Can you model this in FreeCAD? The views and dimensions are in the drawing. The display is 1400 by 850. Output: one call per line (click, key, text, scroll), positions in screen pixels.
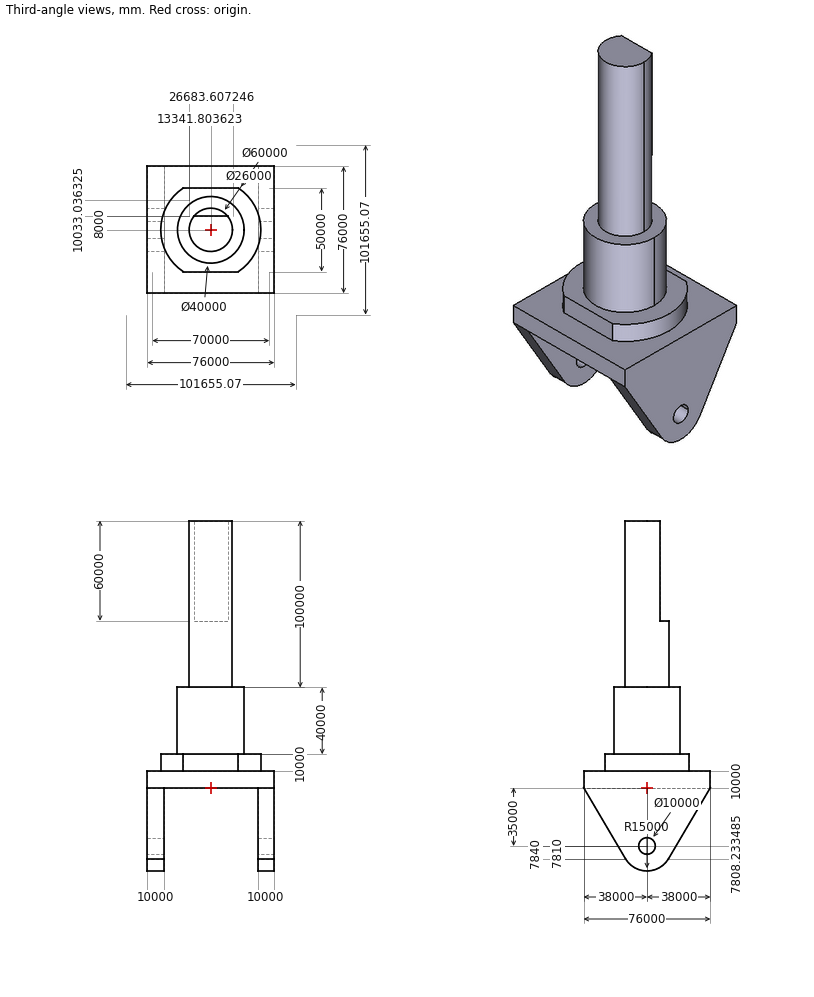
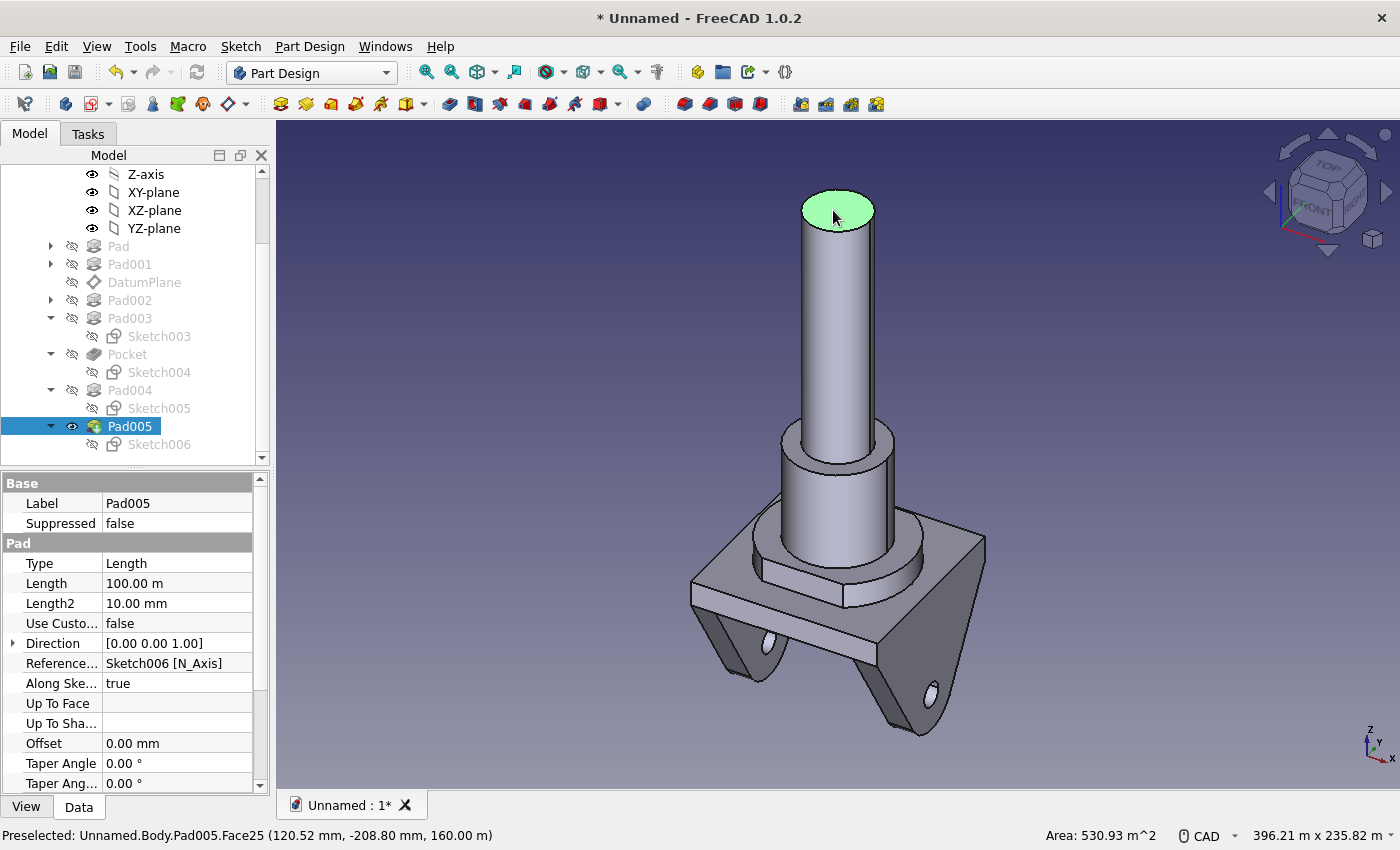
click(90, 104)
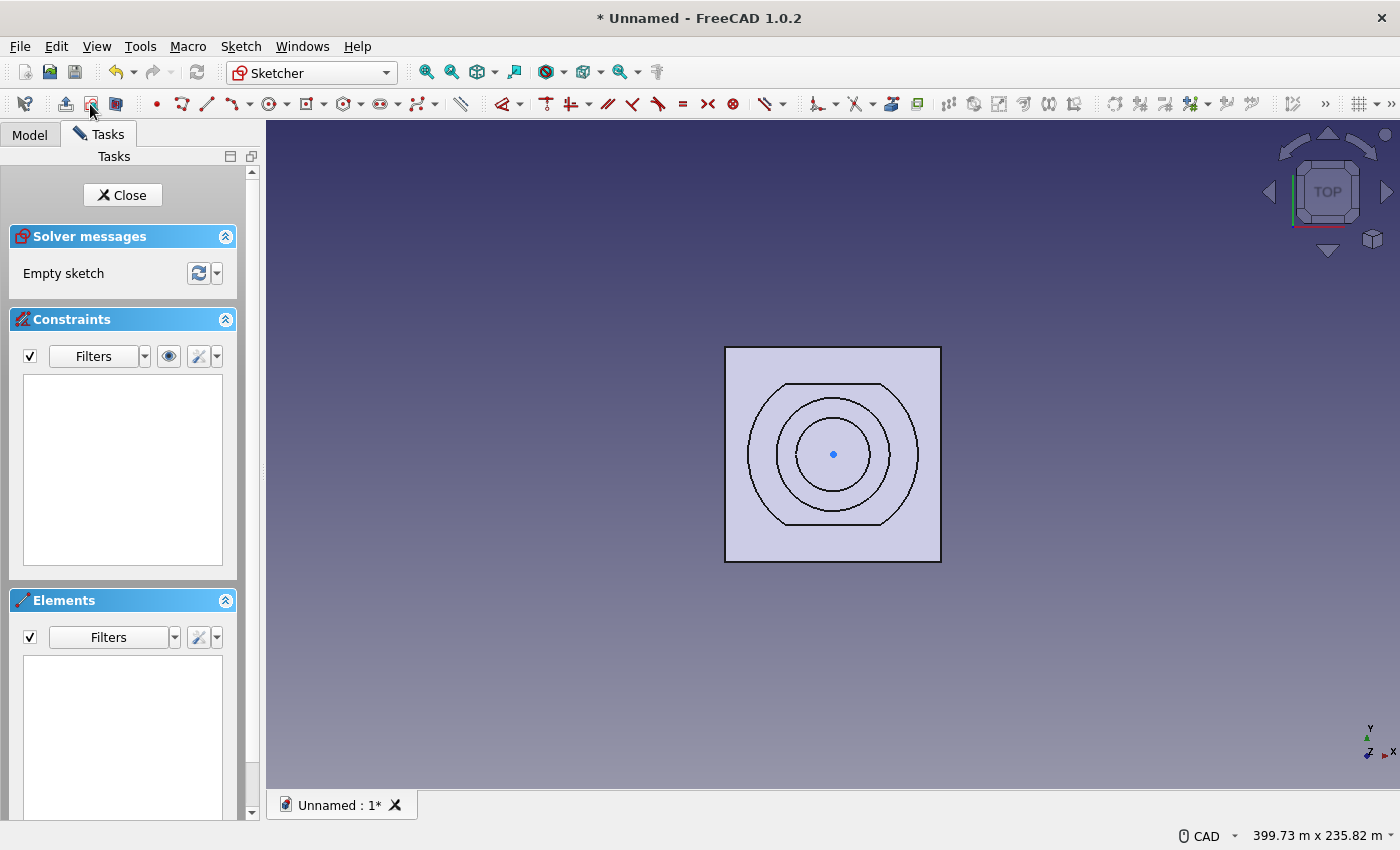
scroll(842, 426, up, 11)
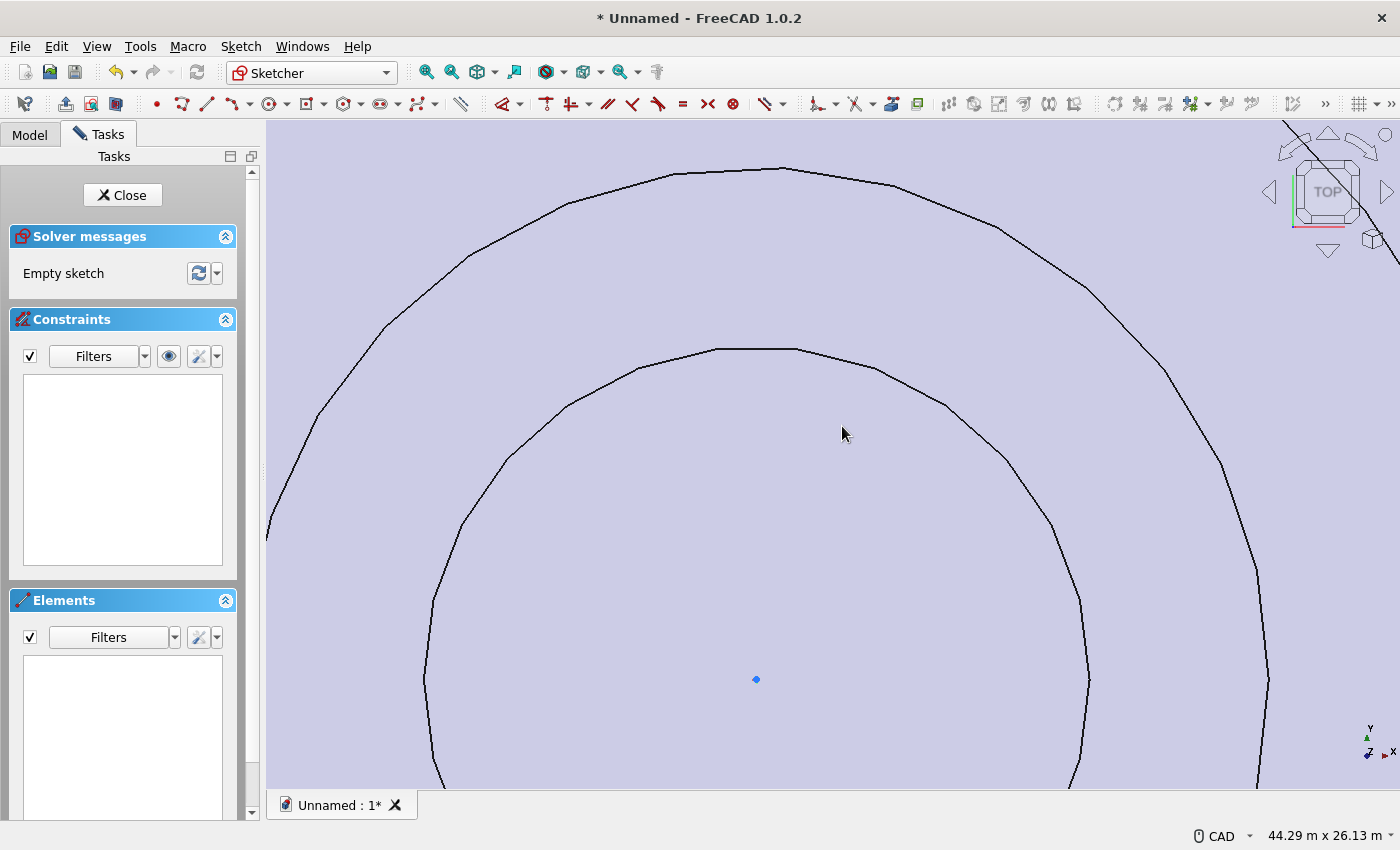
key(g)
key(r)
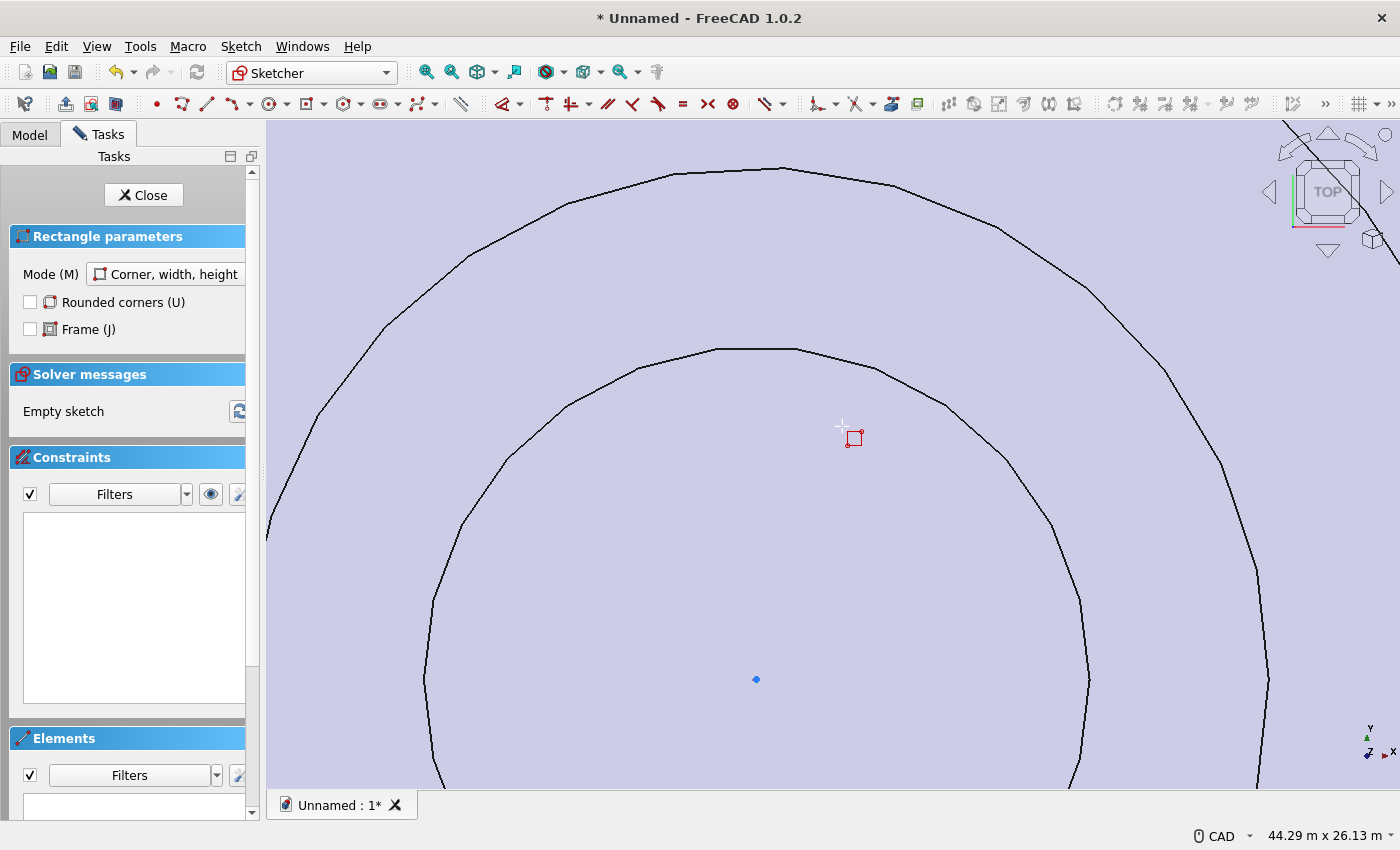
click(415, 218)
click(1098, 475)
key(Escape)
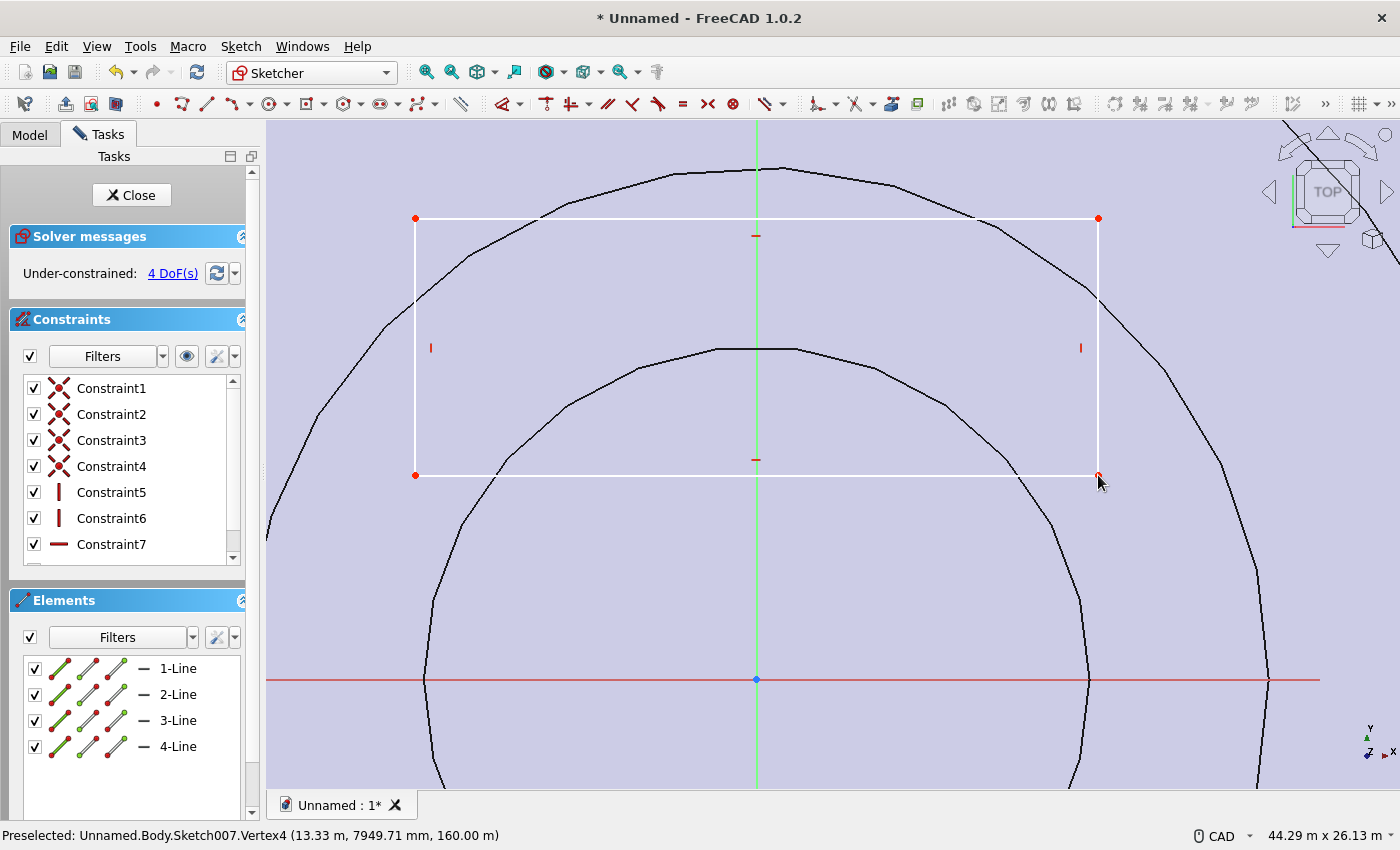
click(502, 104)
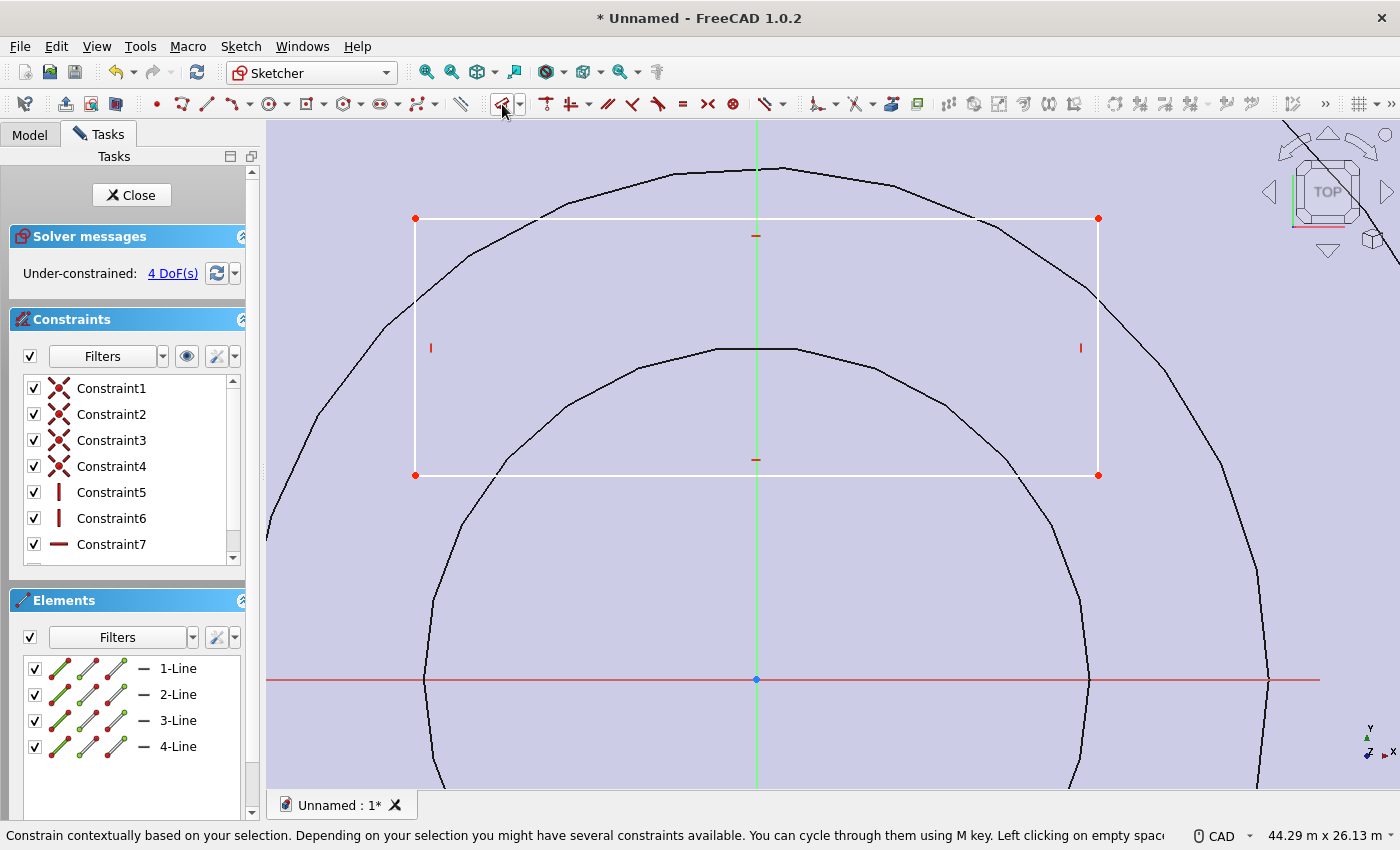
click(415, 476)
click(381, 578)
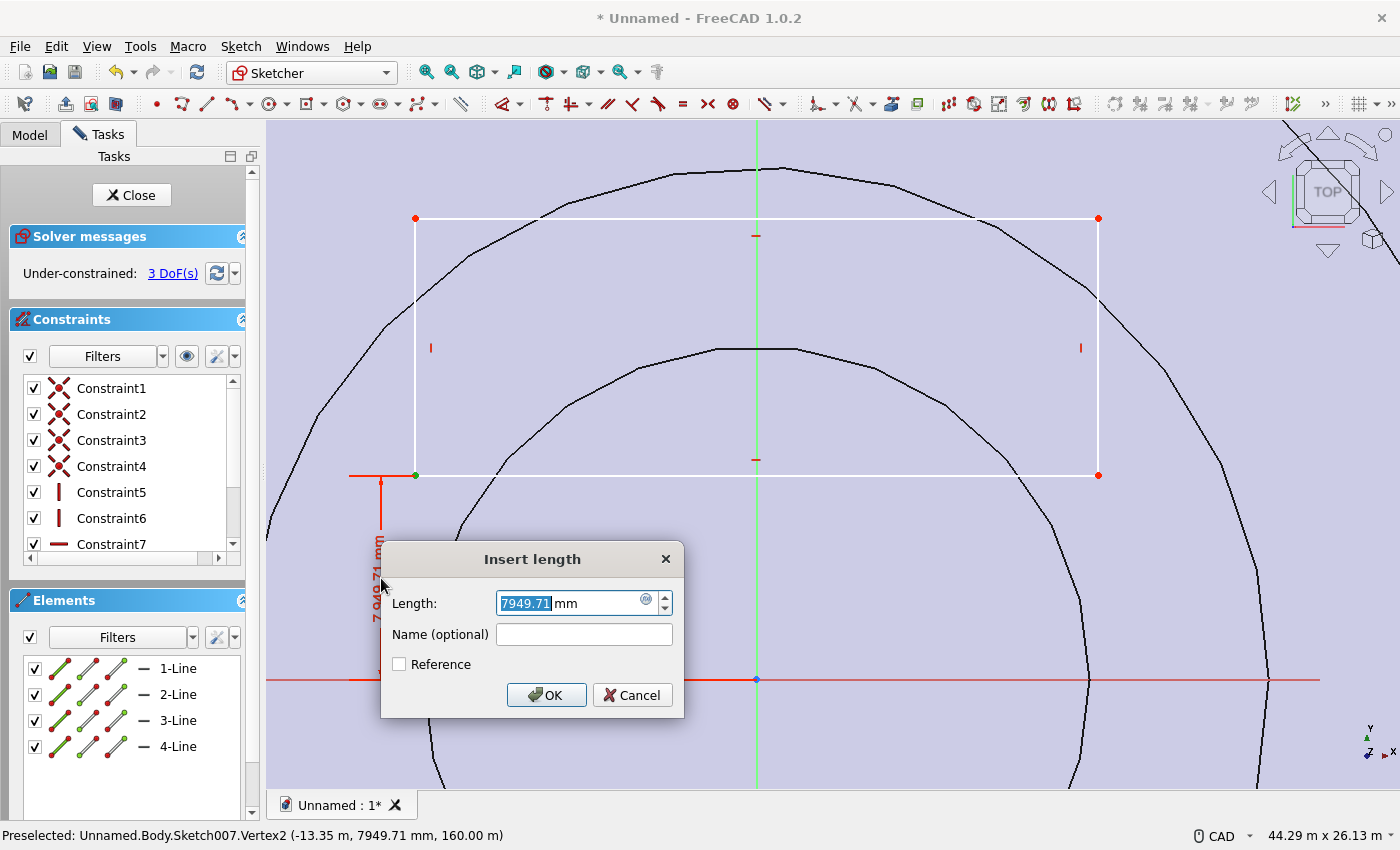
text(8000)
key(Return)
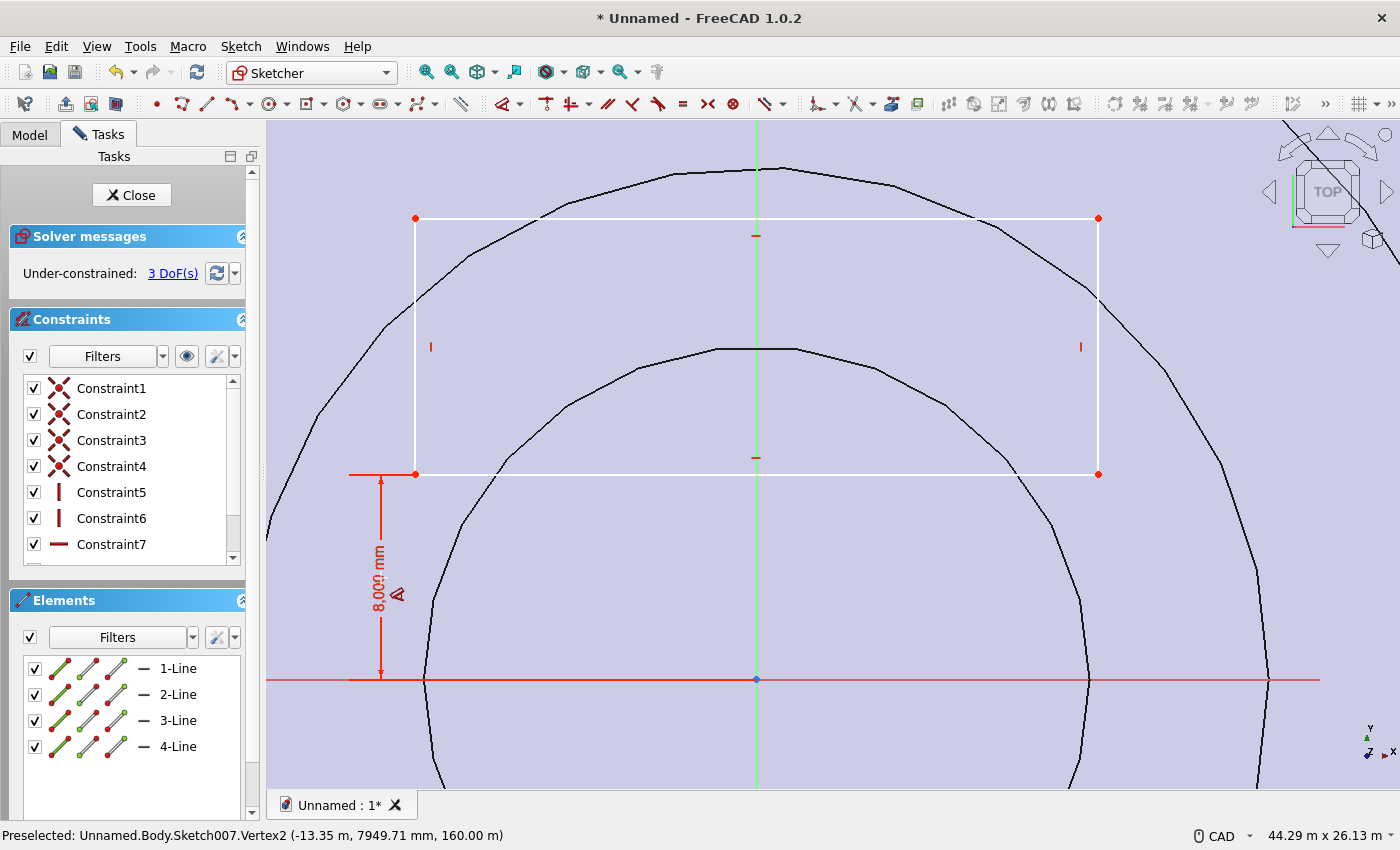
click(415, 296)
click(381, 347)